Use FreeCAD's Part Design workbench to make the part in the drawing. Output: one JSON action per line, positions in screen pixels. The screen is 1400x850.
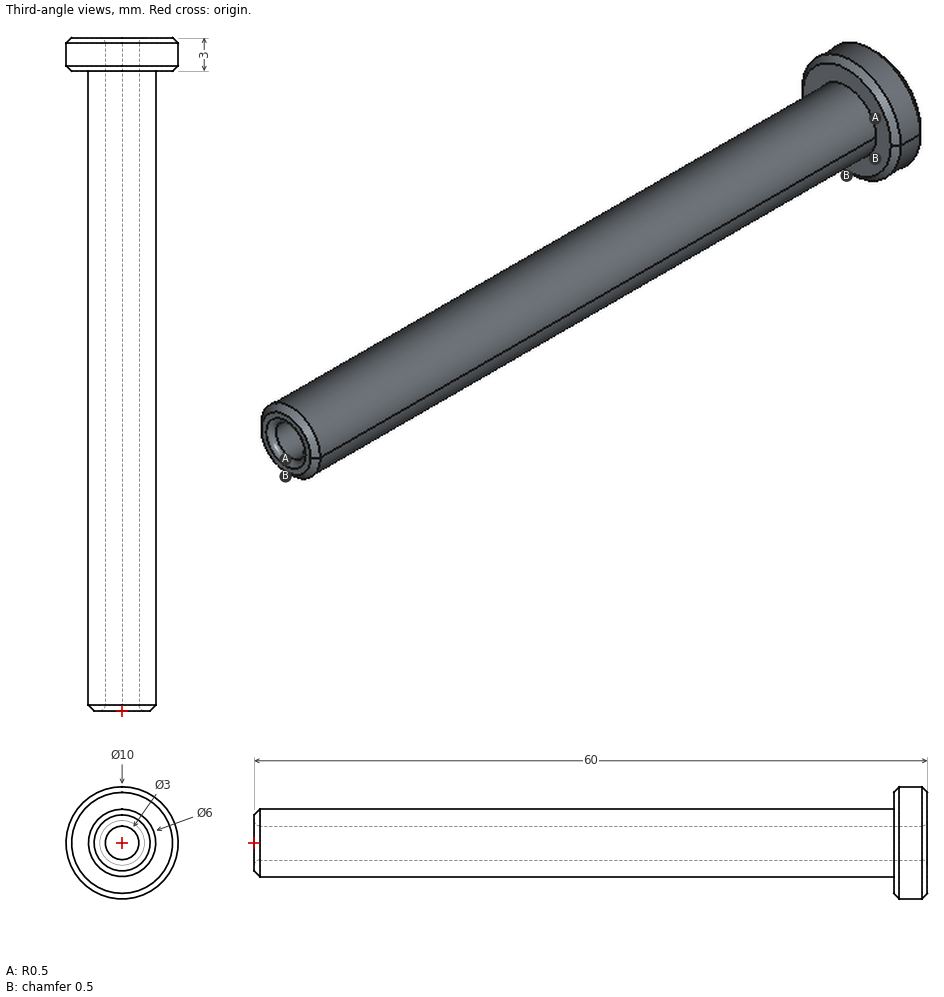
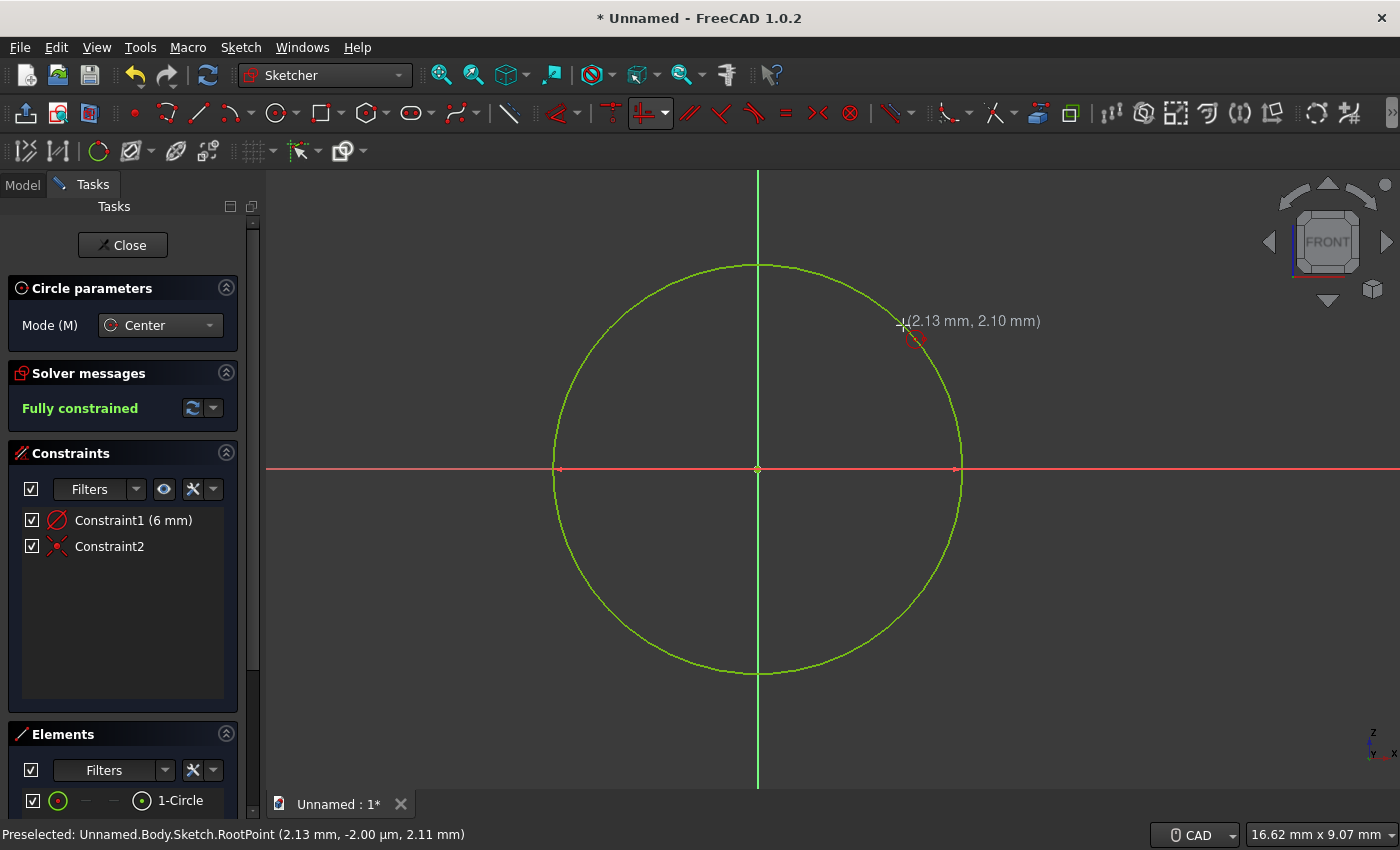
{"action": "left_click", "coordinate": [758, 469]}
{"action": "mouse_move", "coordinate": [830, 397]}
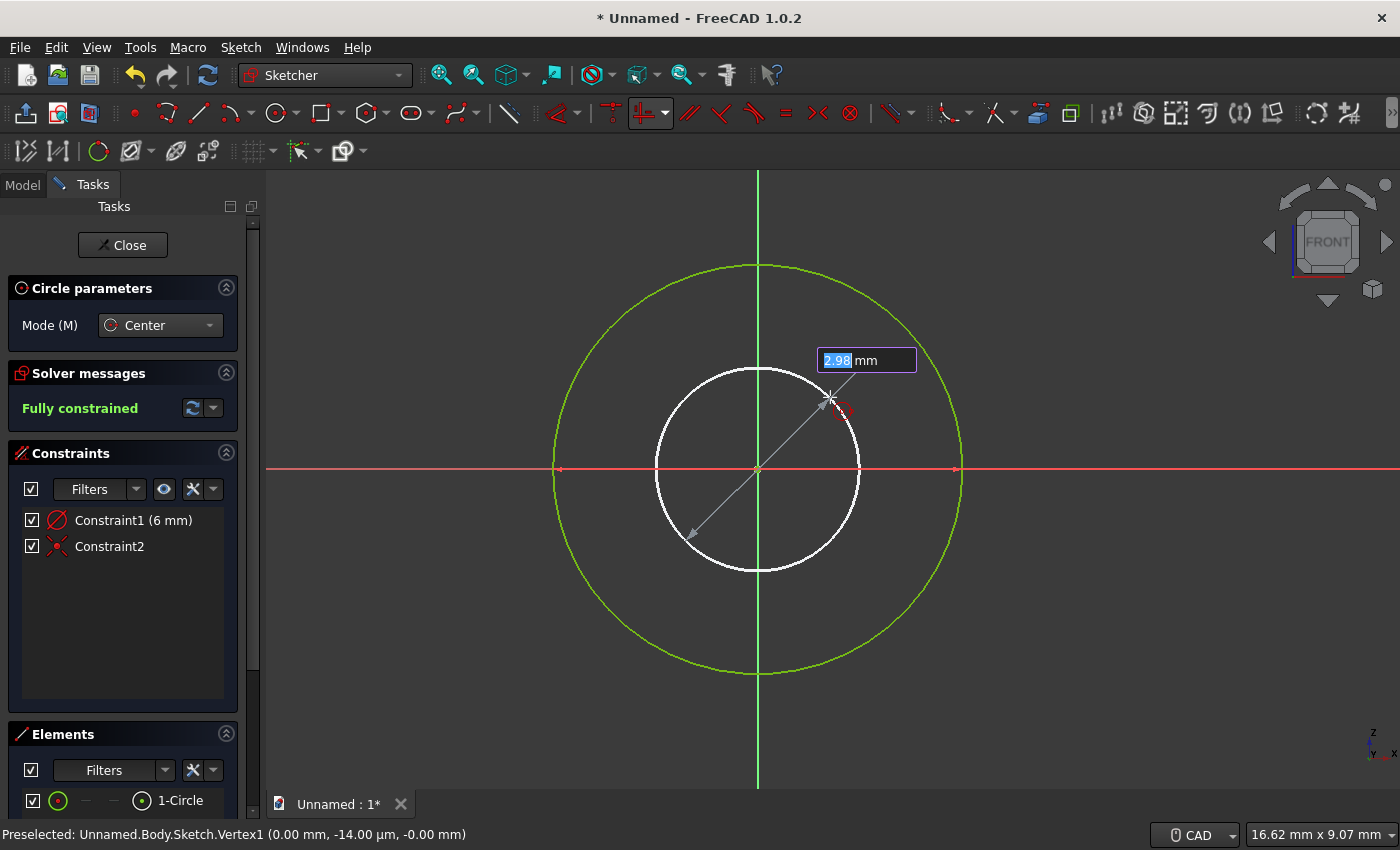
{"action": "type", "text": "3"}
{"action": "key", "text": "Return"}
{"action": "key", "text": "Escape"}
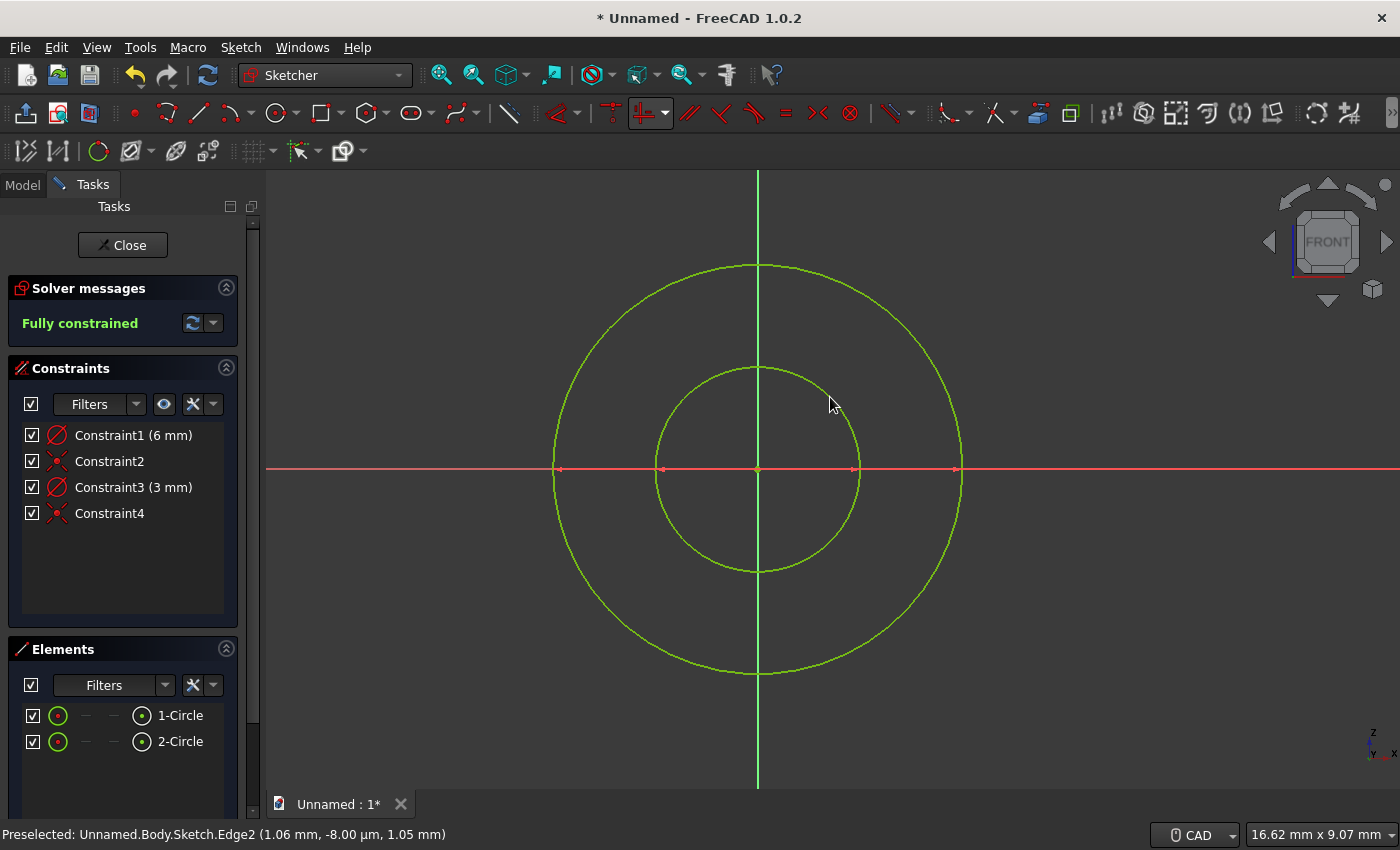
{"action": "left_click", "coordinate": [123, 245]}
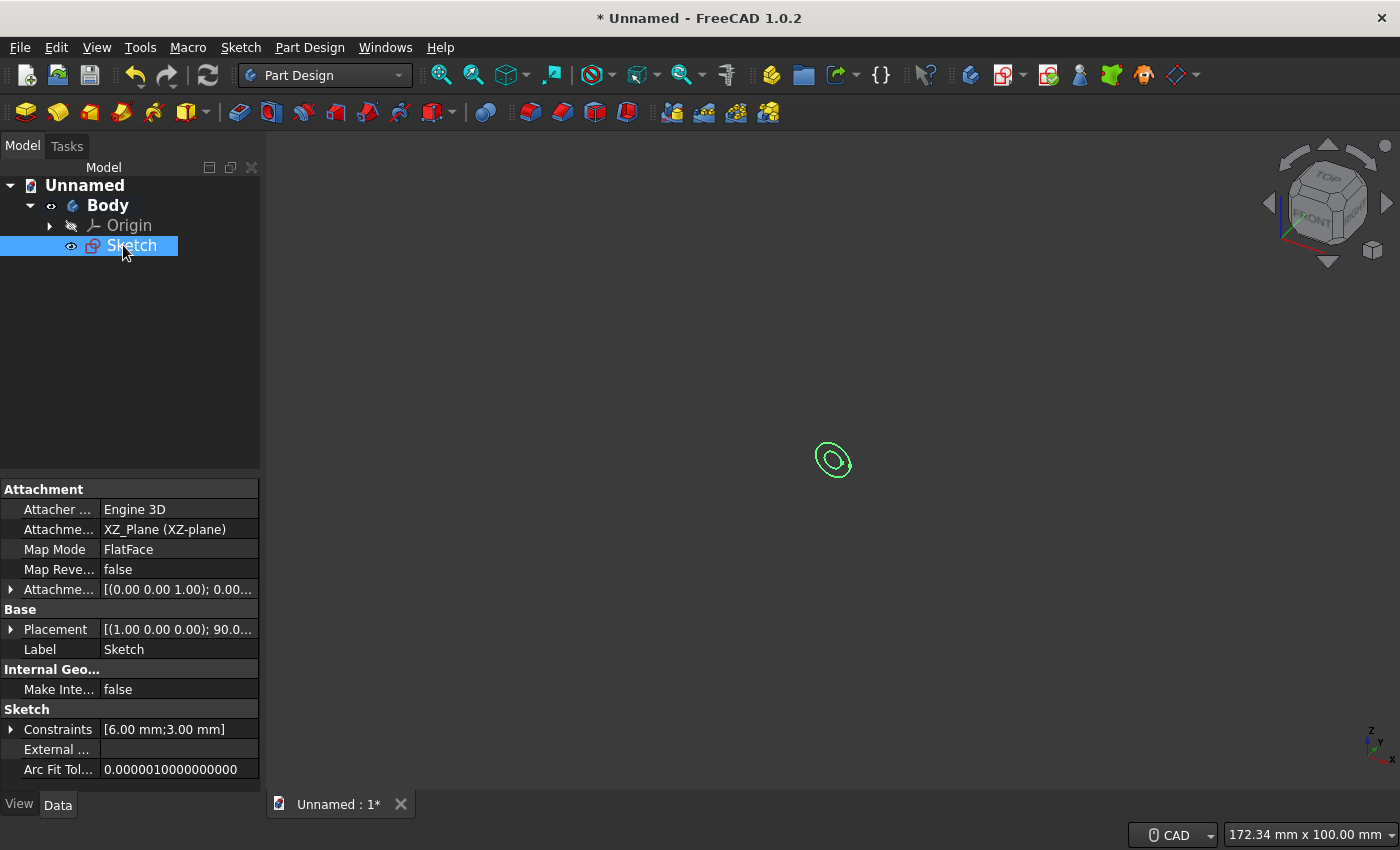
{"action": "left_click", "coordinate": [26, 112]}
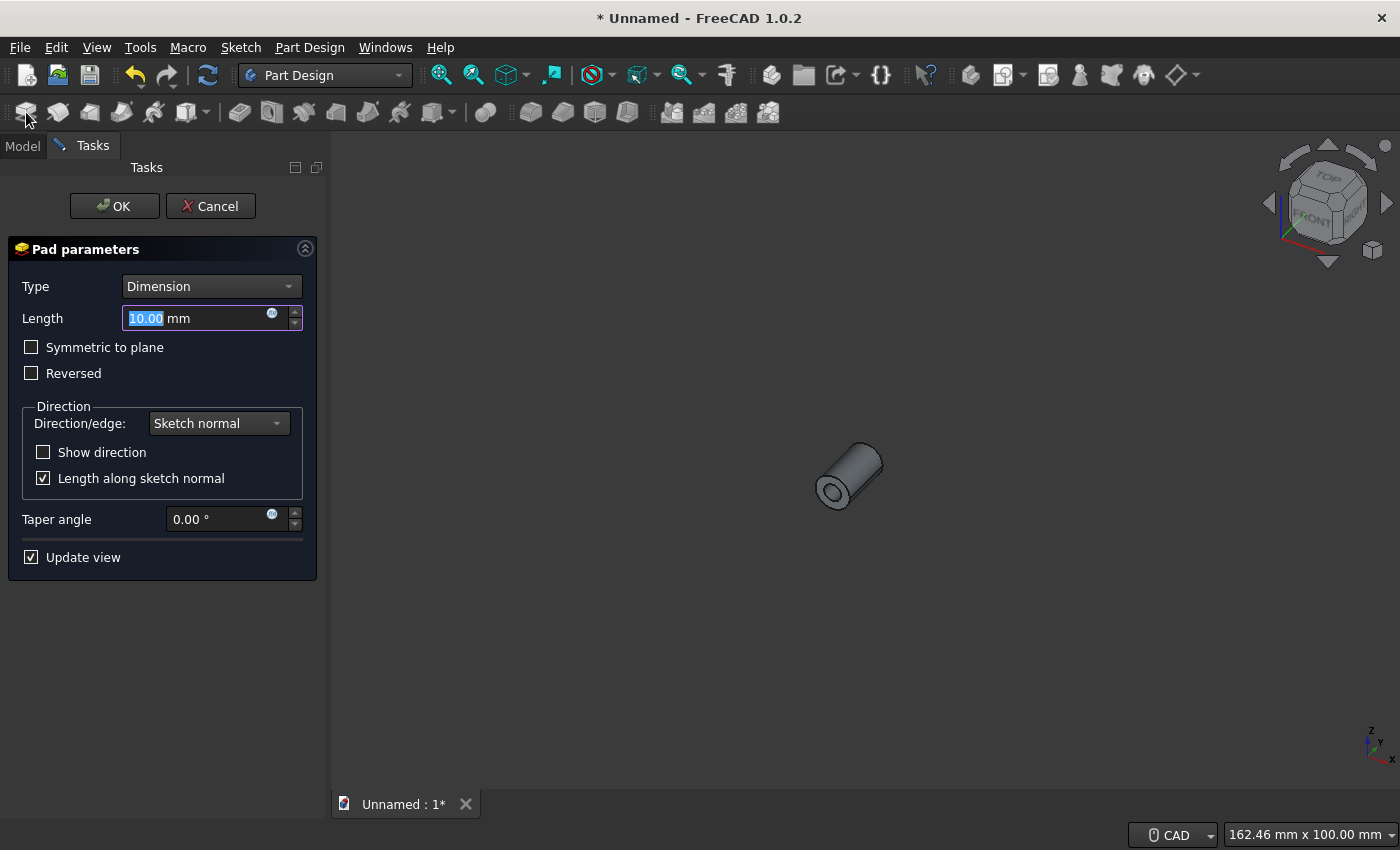
{"action": "type", "text": "60"}
{"action": "key", "text": "Tab"}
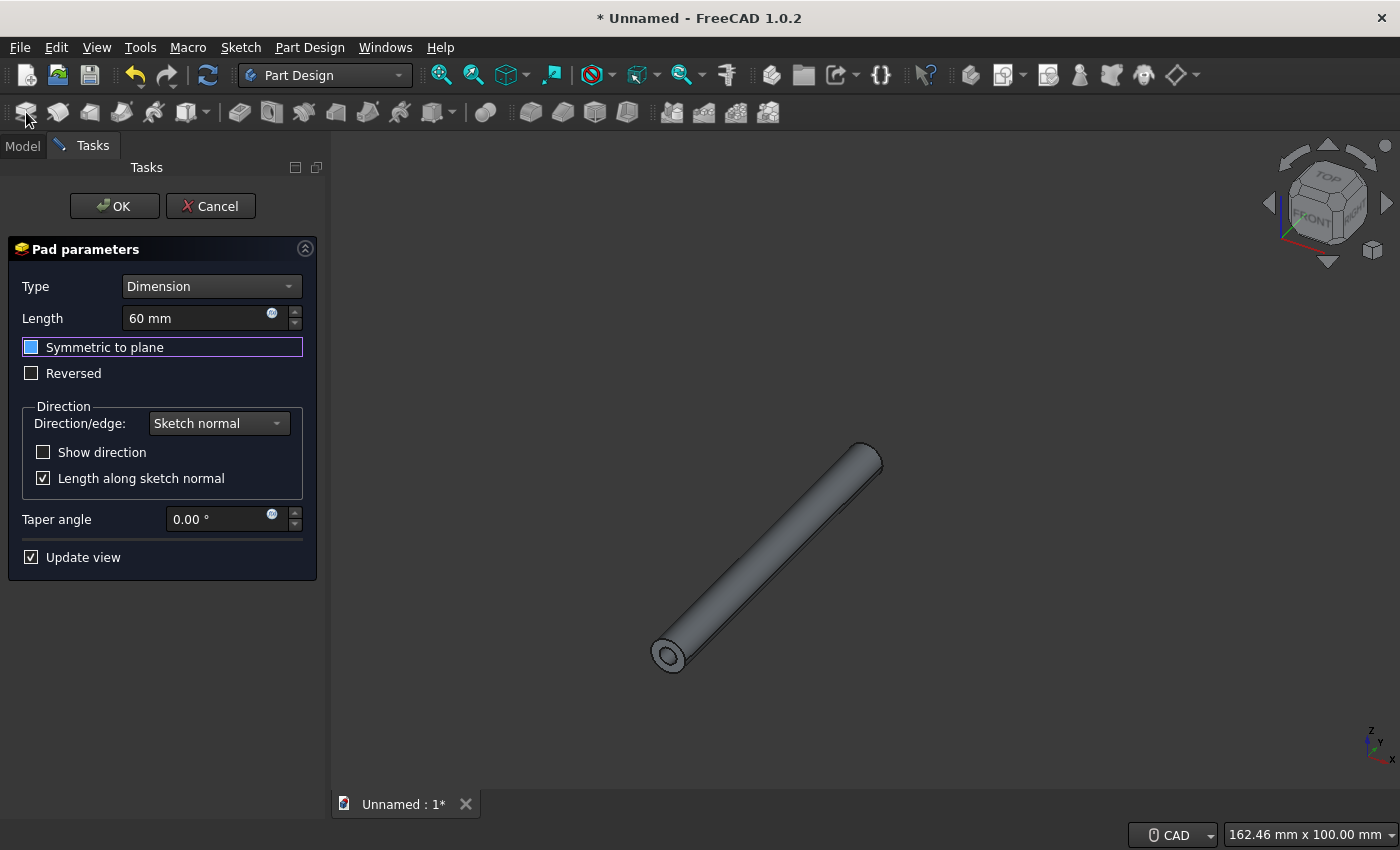
{"action": "left_click", "coordinate": [30, 373]}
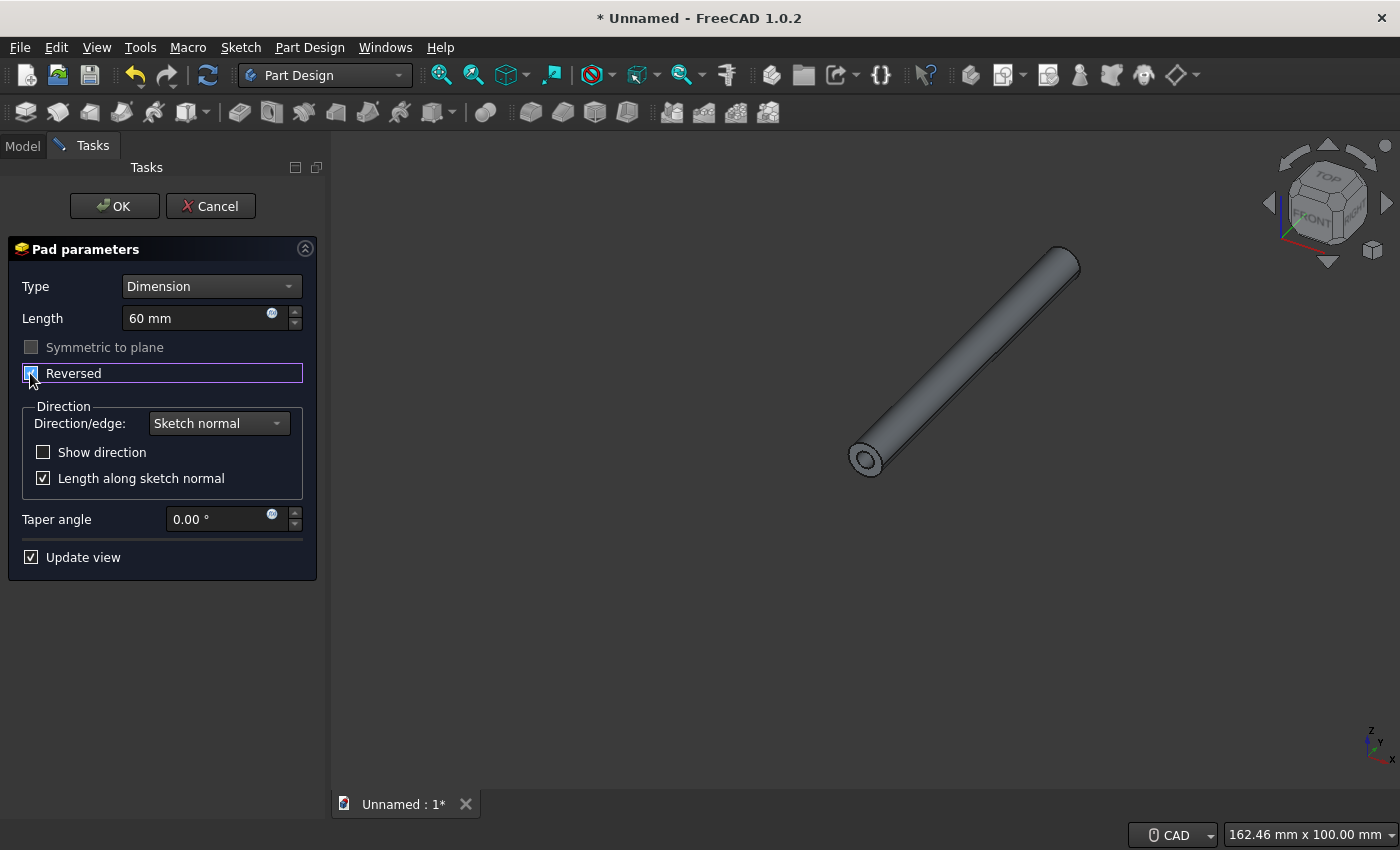
{"action": "left_click", "coordinate": [115, 206]}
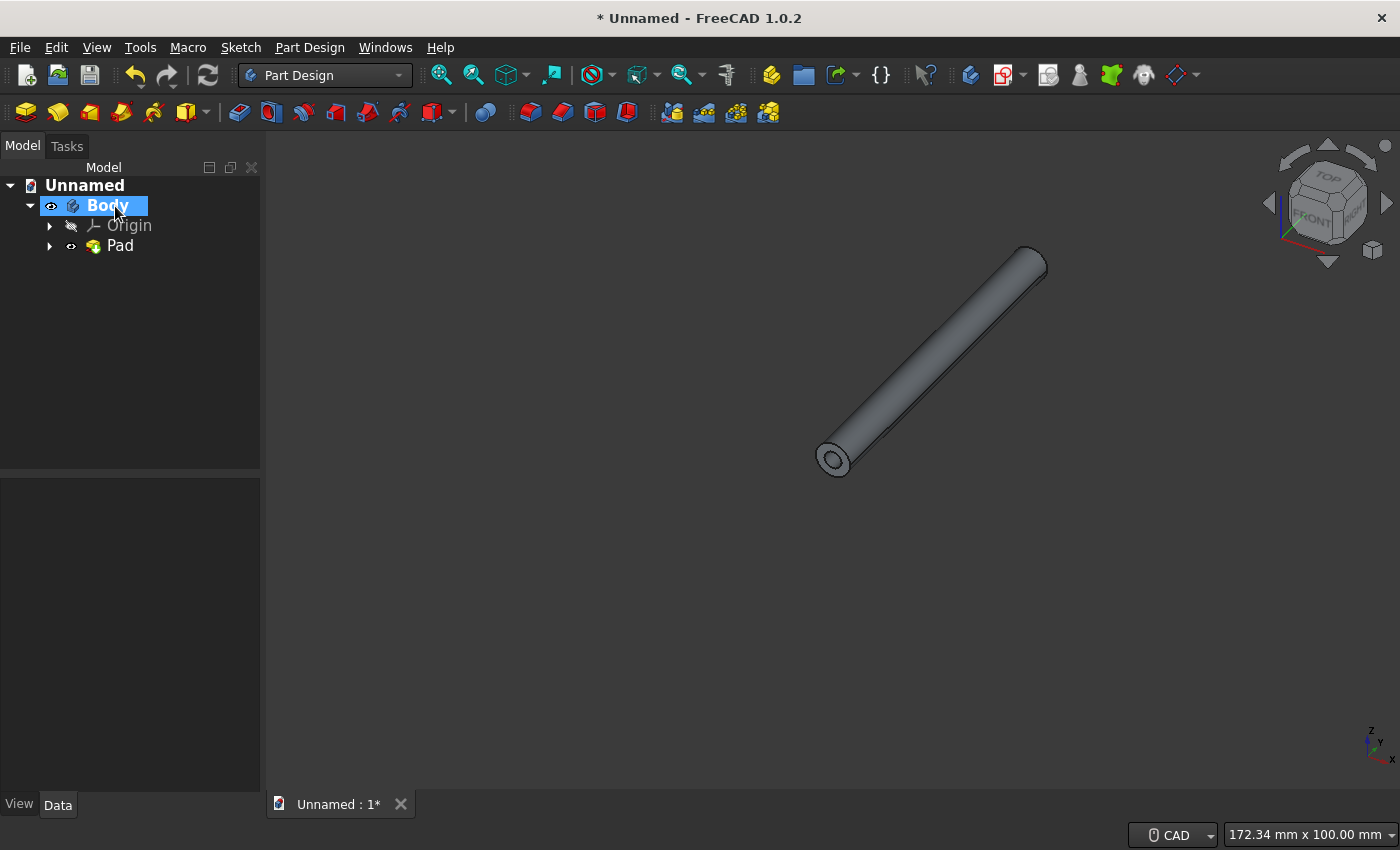
{"action": "key", "text": "v f"}